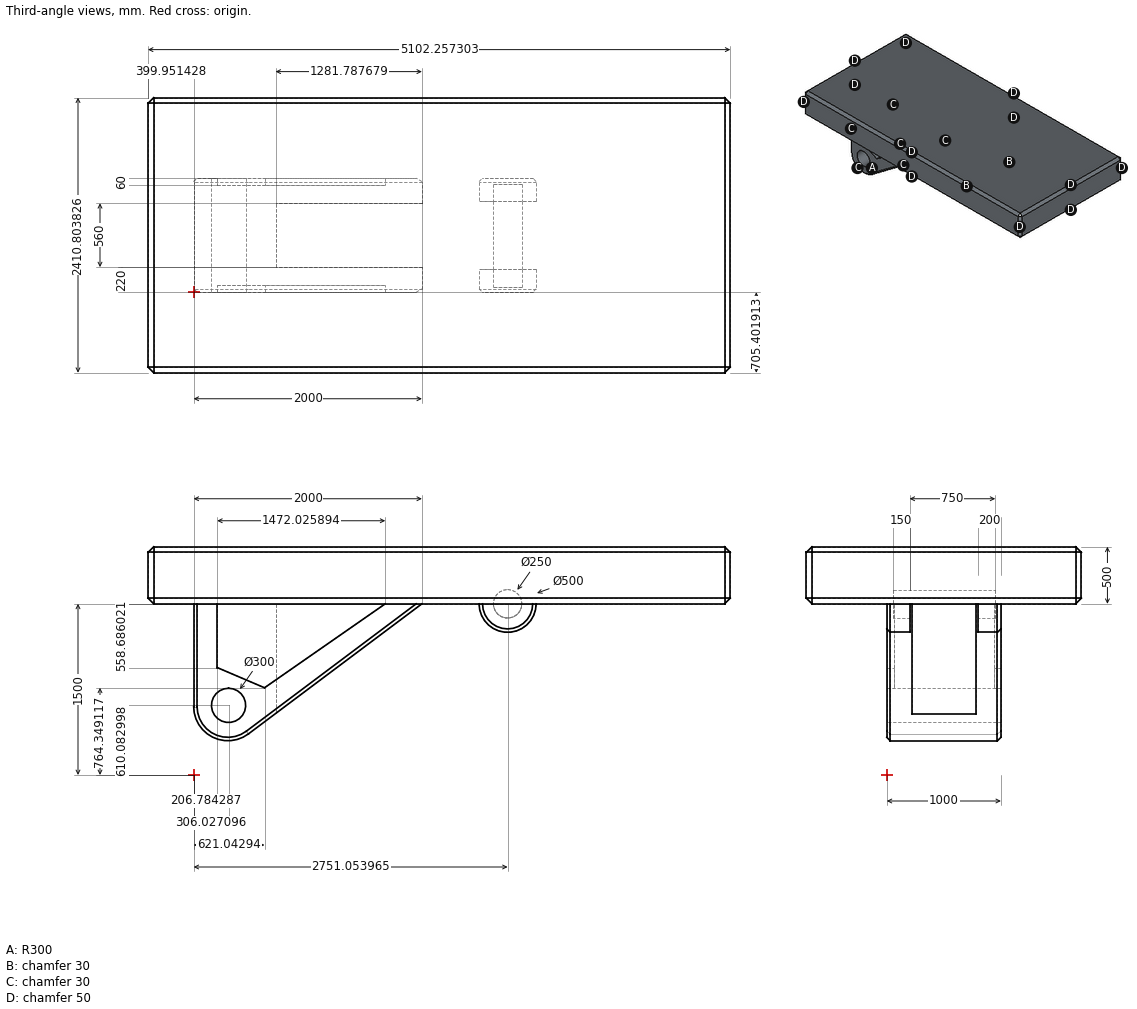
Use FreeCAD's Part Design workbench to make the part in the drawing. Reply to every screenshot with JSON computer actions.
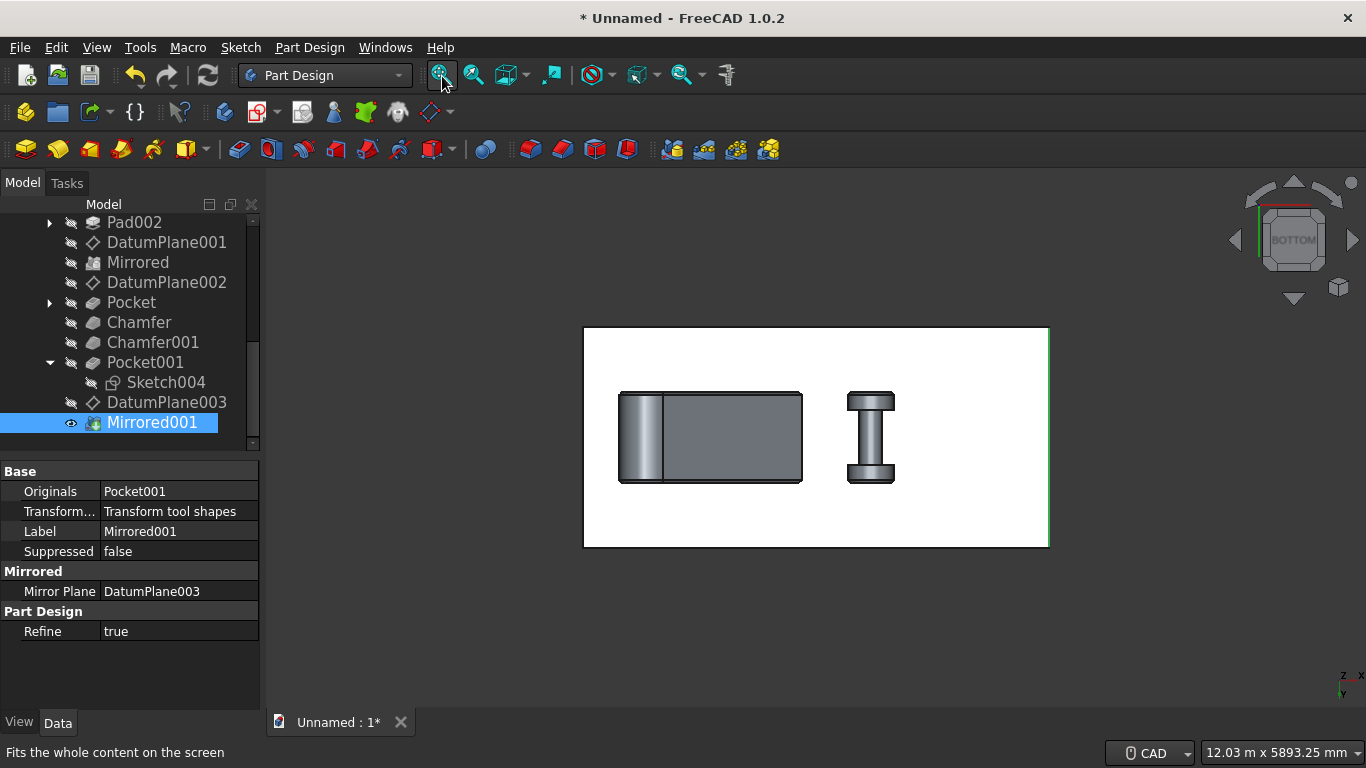
{"action": "left_click", "coordinate": [583, 436], "text": "ctrl"}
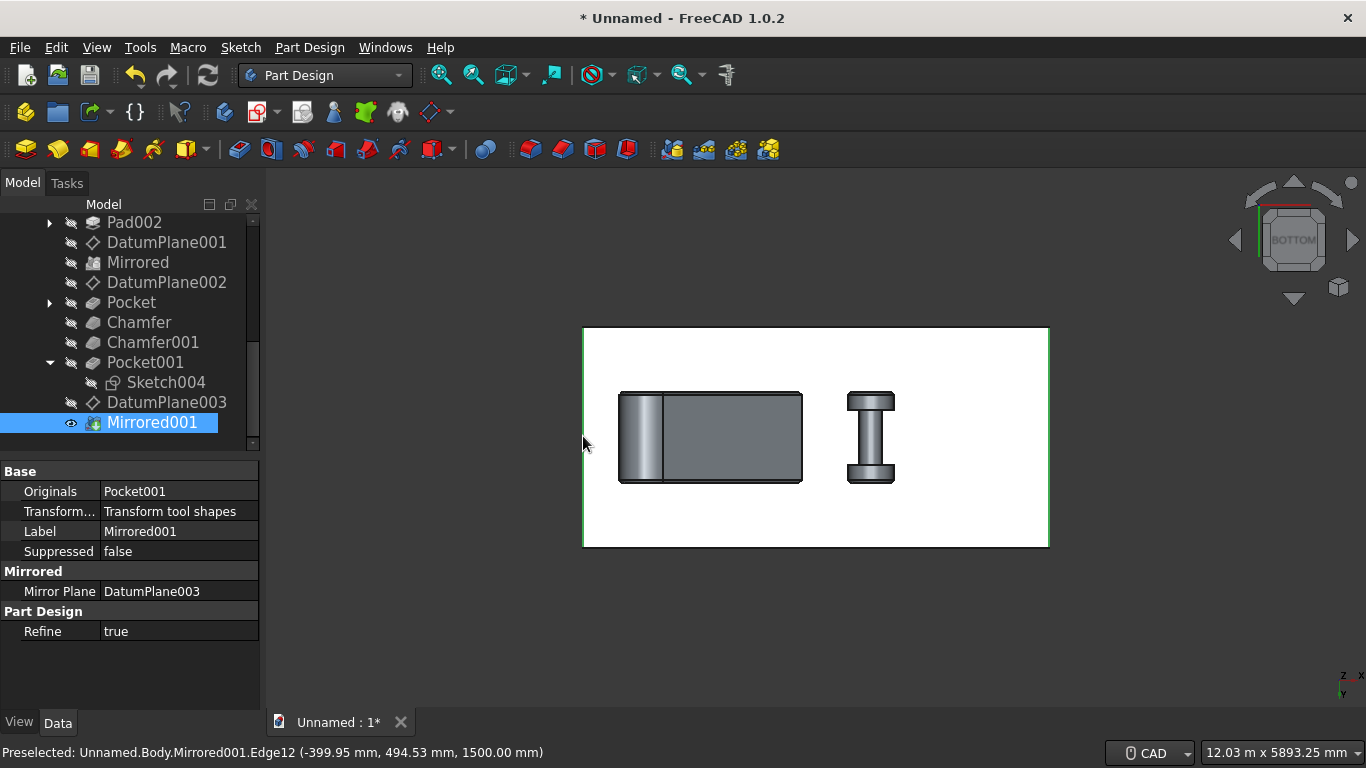
{"action": "left_click", "coordinate": [564, 150]}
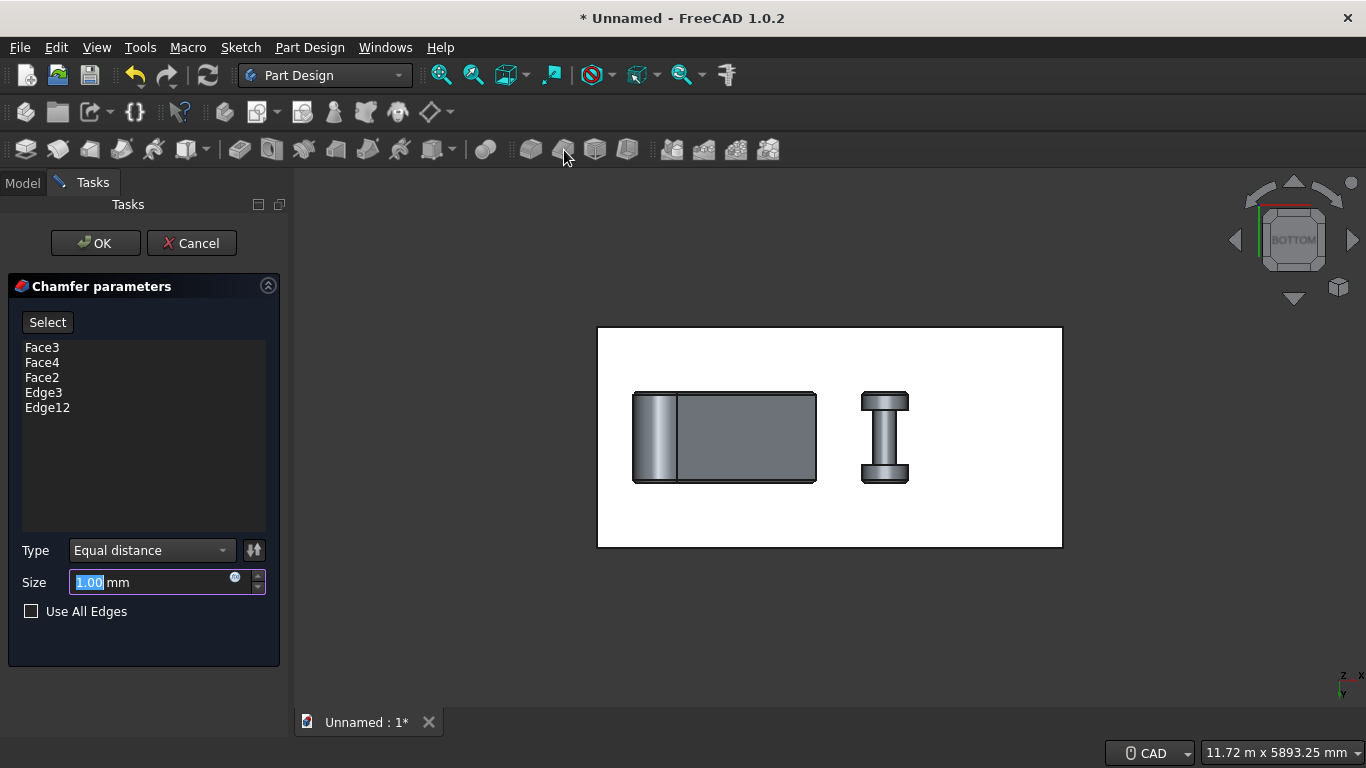
{"action": "type", "text": "50"}
{"action": "key", "text": "Tab"}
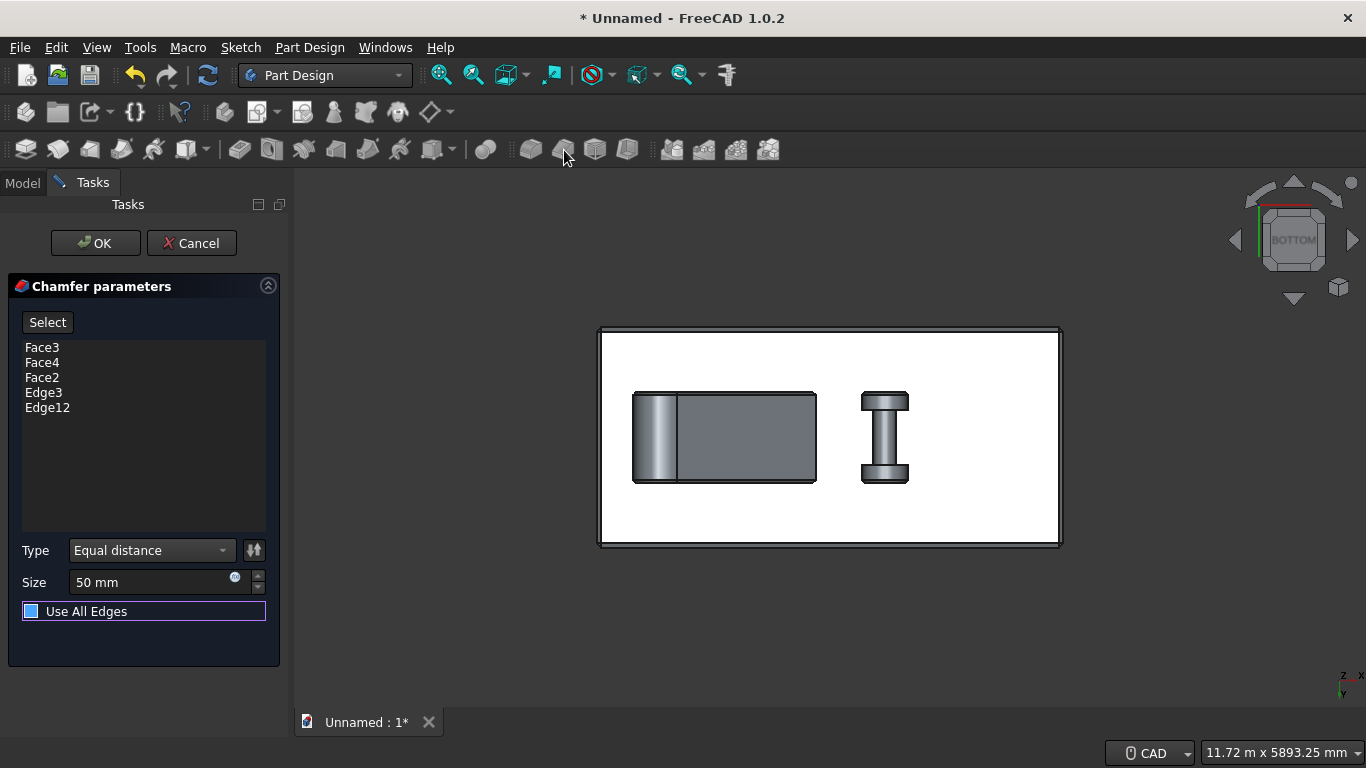
{"action": "left_click", "coordinate": [96, 243]}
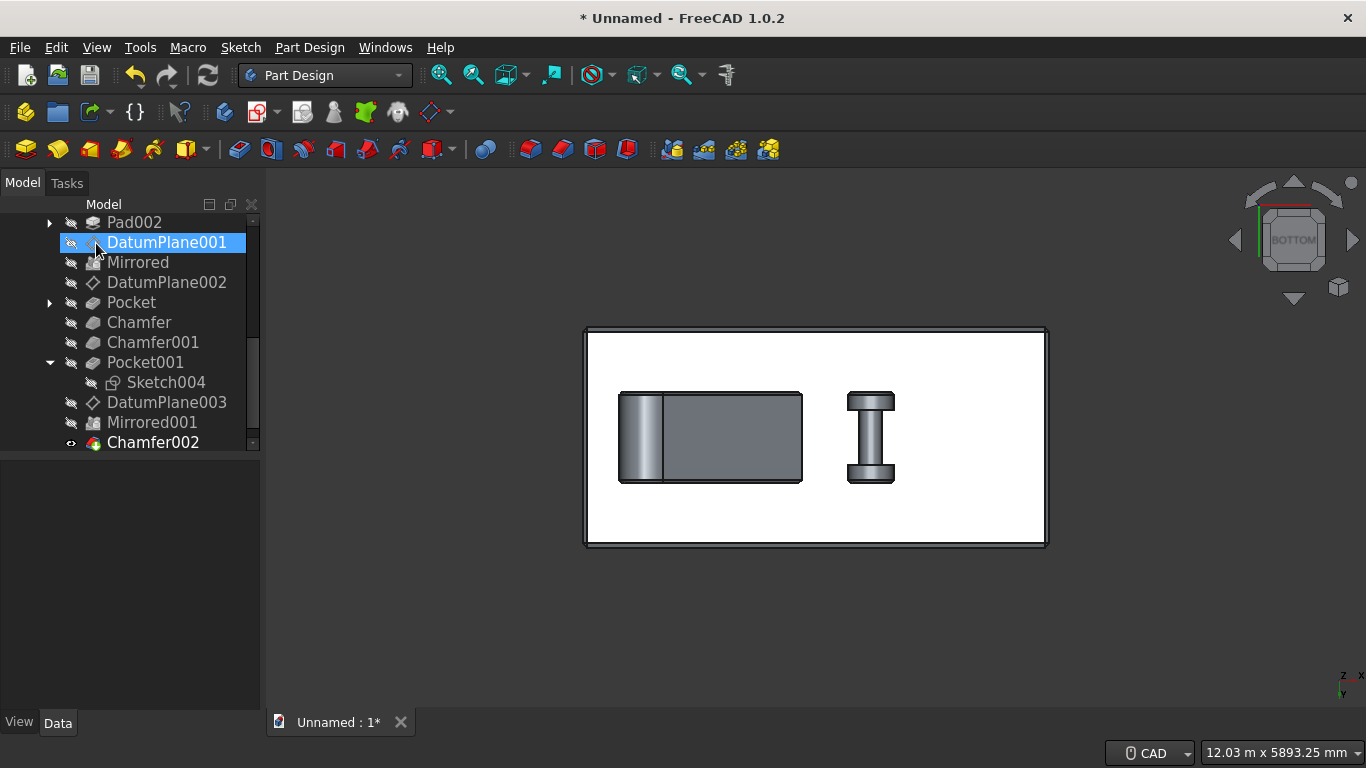
{"action": "left_click", "coordinate": [442, 76]}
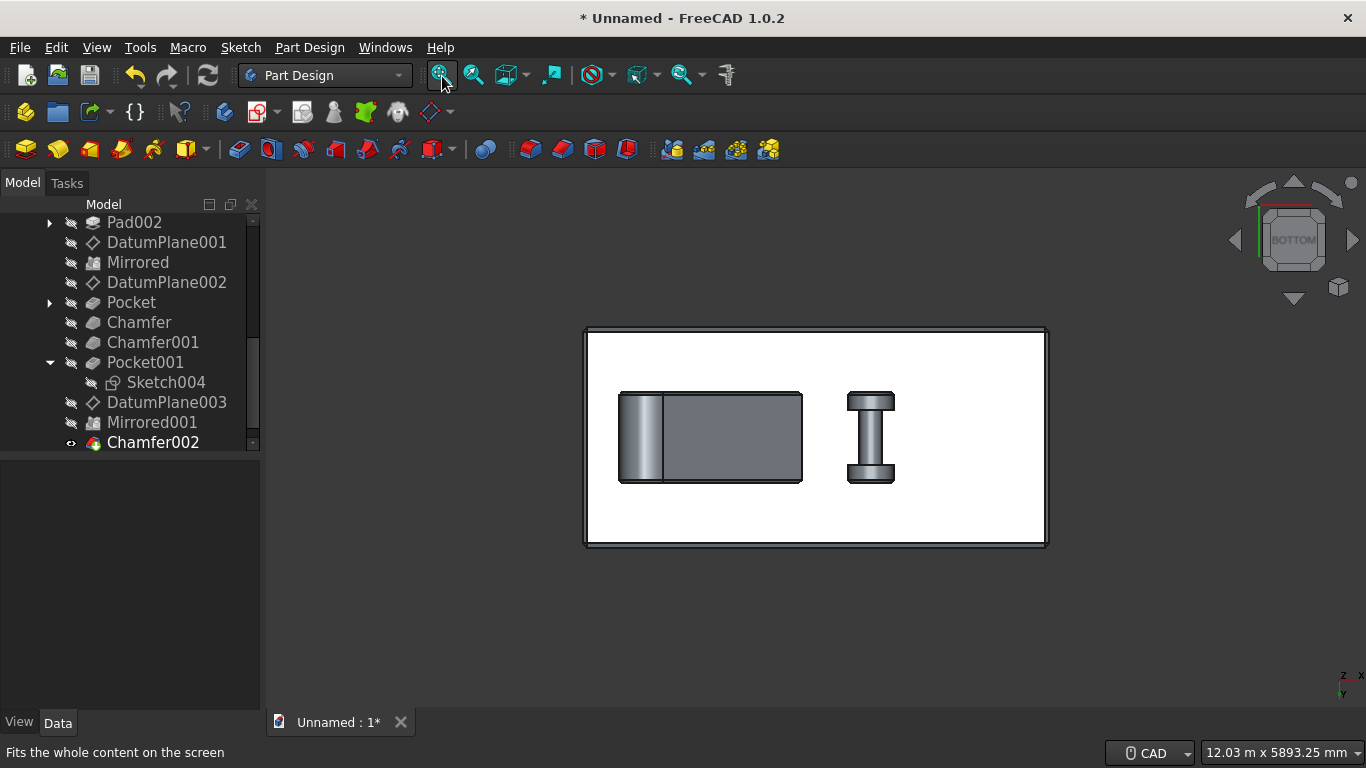
{"action": "left_click", "coordinate": [947, 436]}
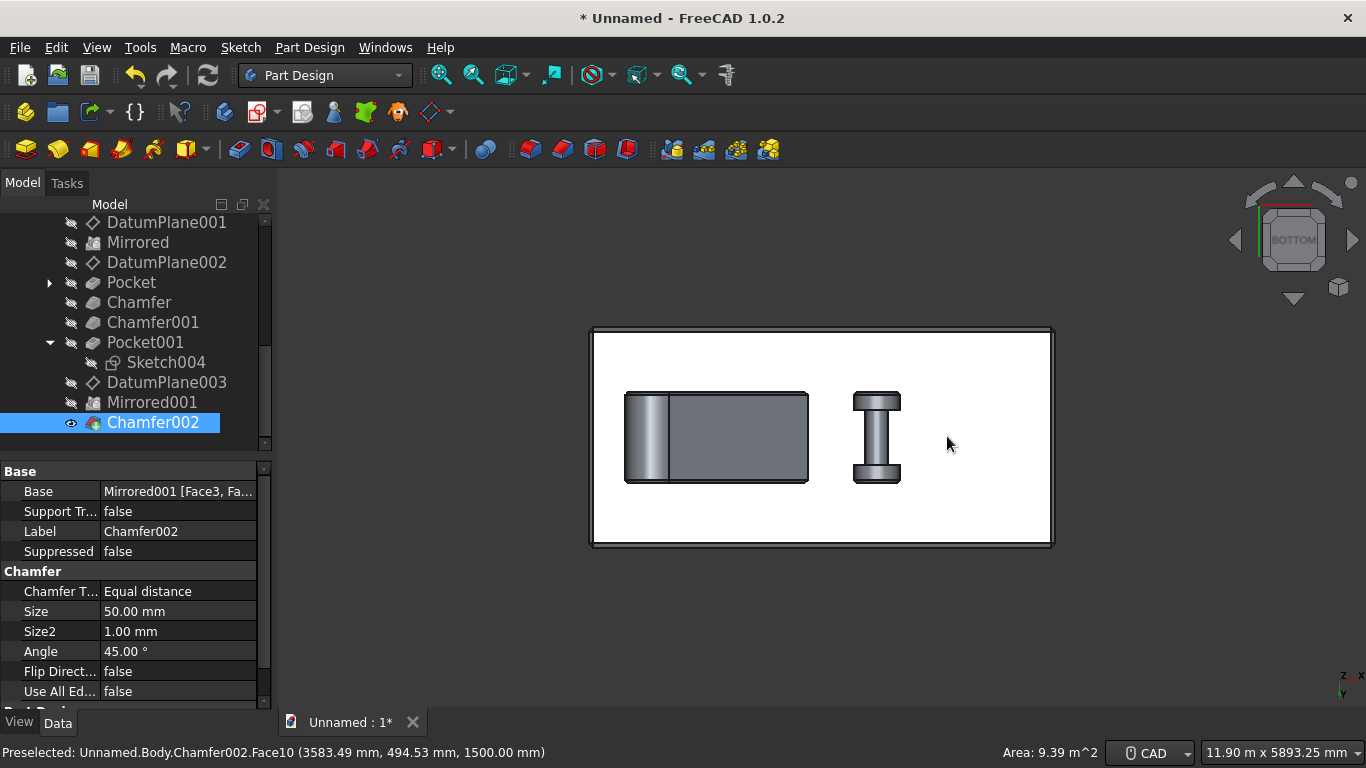
{"action": "left_click", "coordinate": [258, 112]}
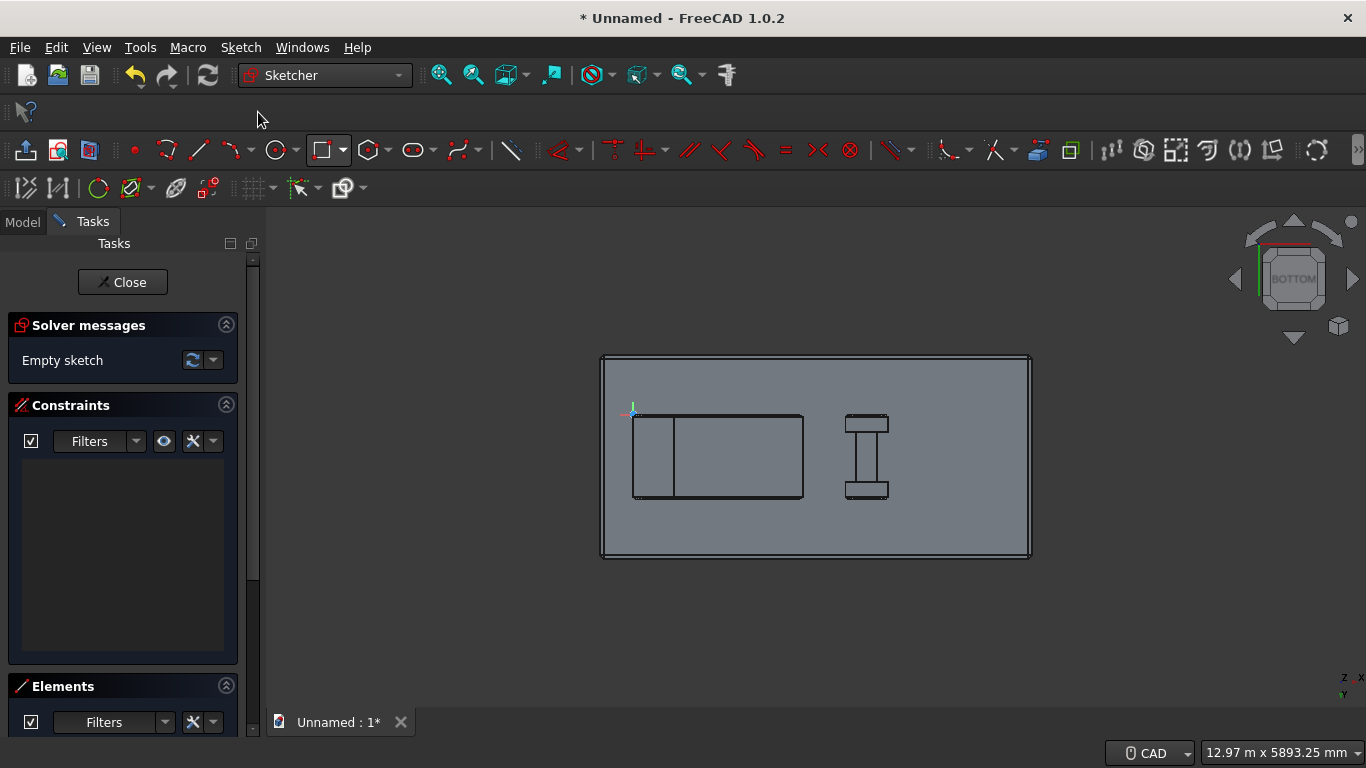
{"action": "left_click", "coordinate": [90, 150]}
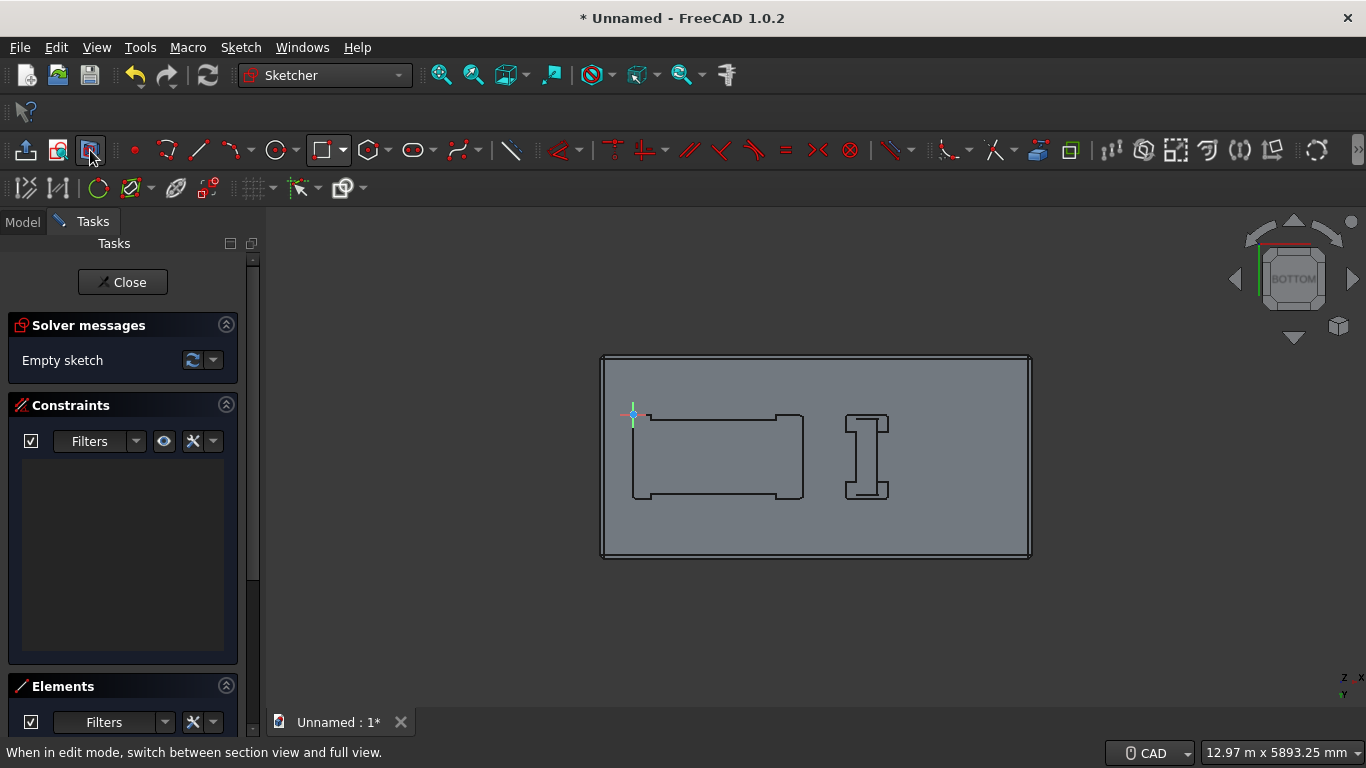
{"action": "scroll", "coordinate": [709, 445], "scroll_direction": "up", "scroll_amount": 7}